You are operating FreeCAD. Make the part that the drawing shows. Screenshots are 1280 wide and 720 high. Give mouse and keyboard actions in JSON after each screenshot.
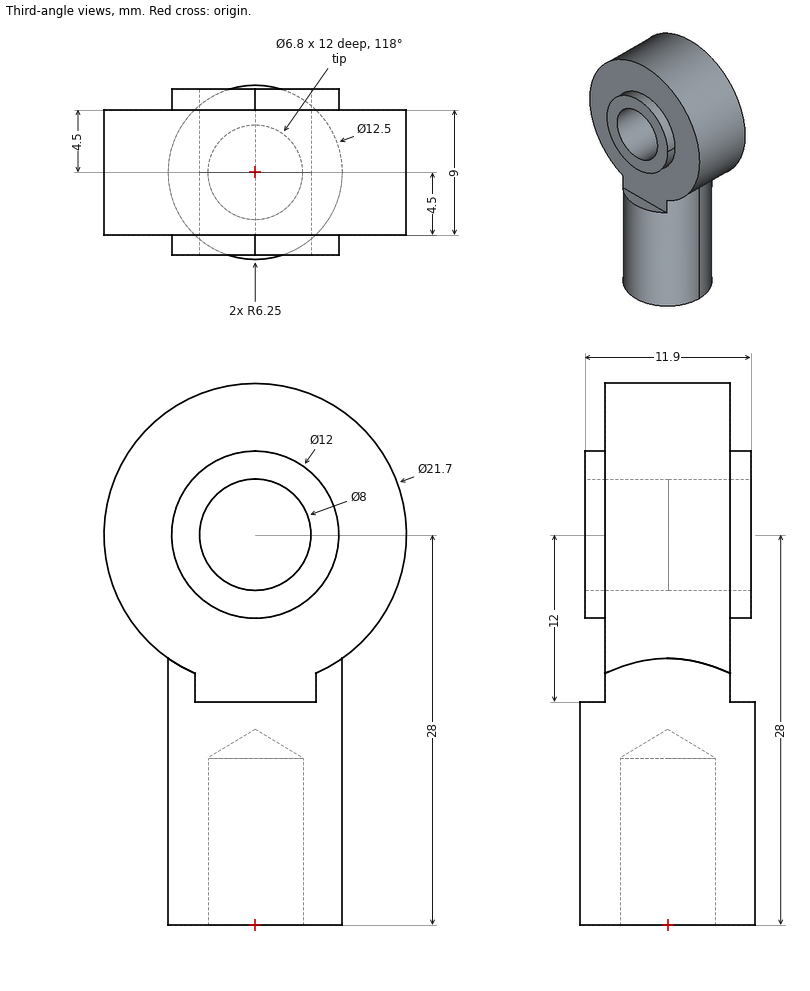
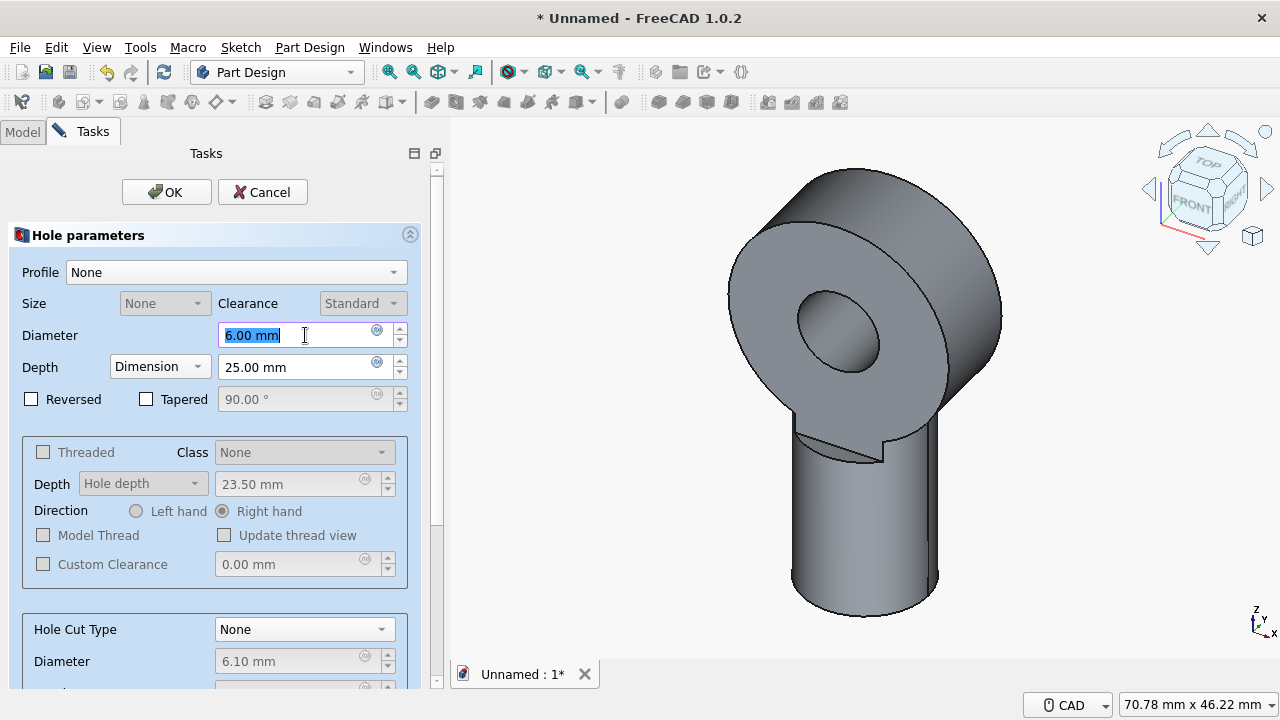
{"action": "type", "text": "6.8"}
{"action": "key", "text": "Tab"}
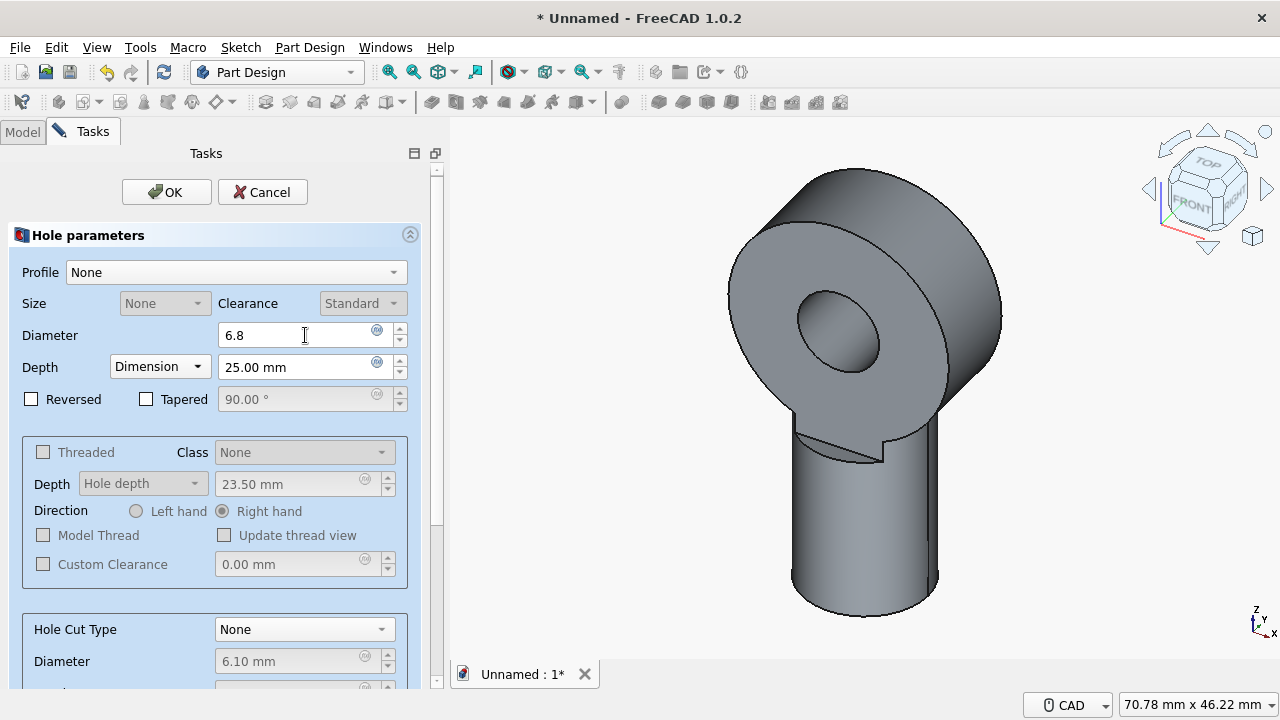
{"action": "triple_click", "coordinate": [305, 367]}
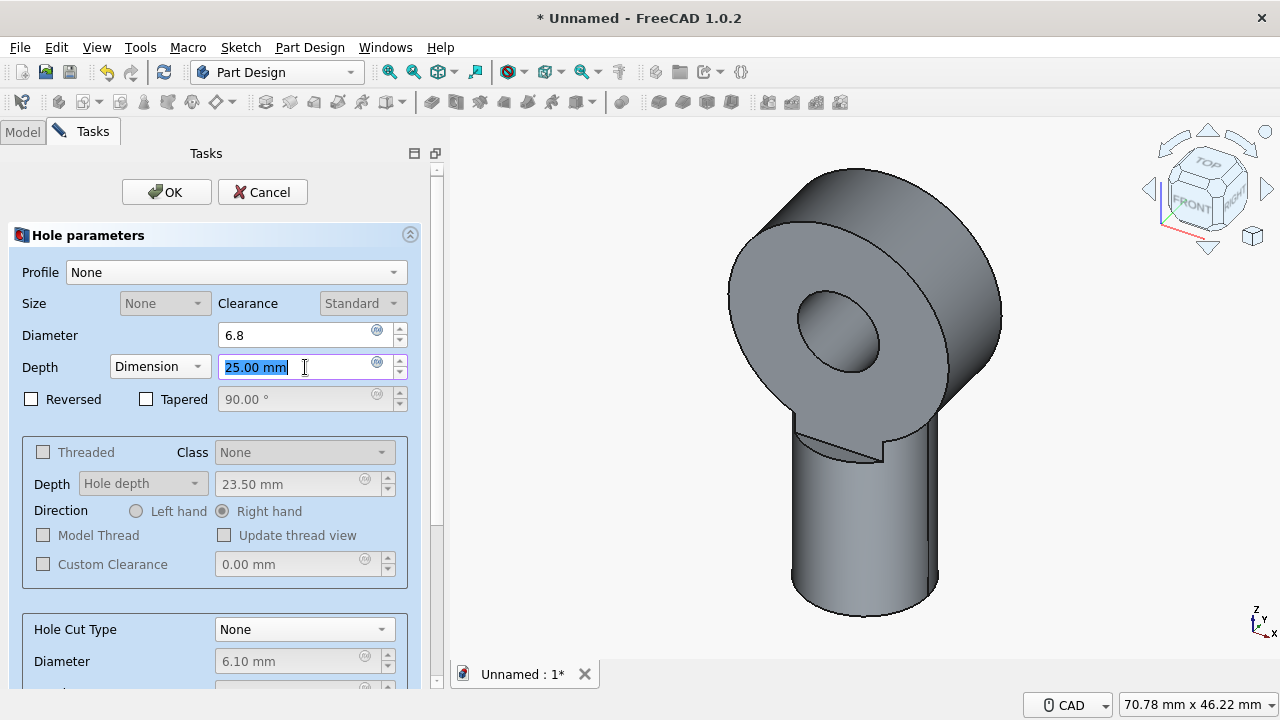
{"action": "type", "text": "12"}
{"action": "key", "text": "Tab"}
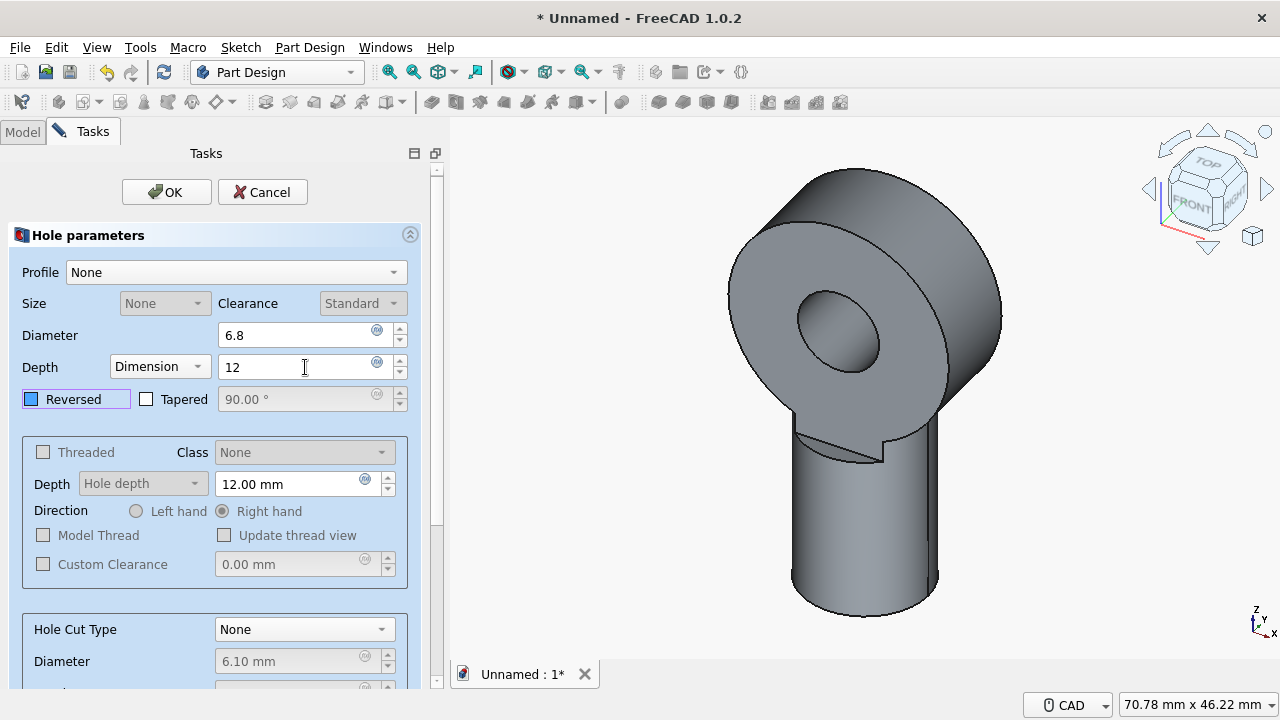
{"action": "left_click", "coordinate": [30, 399]}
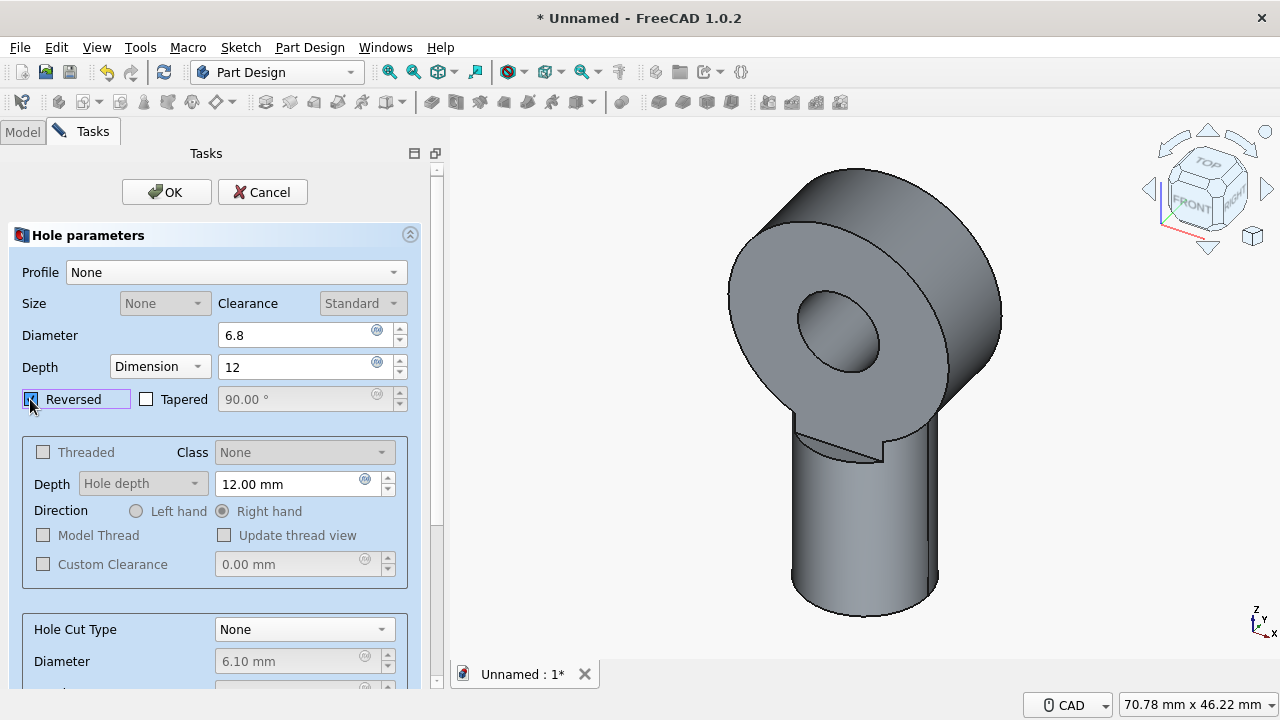
{"action": "left_click", "coordinate": [167, 192]}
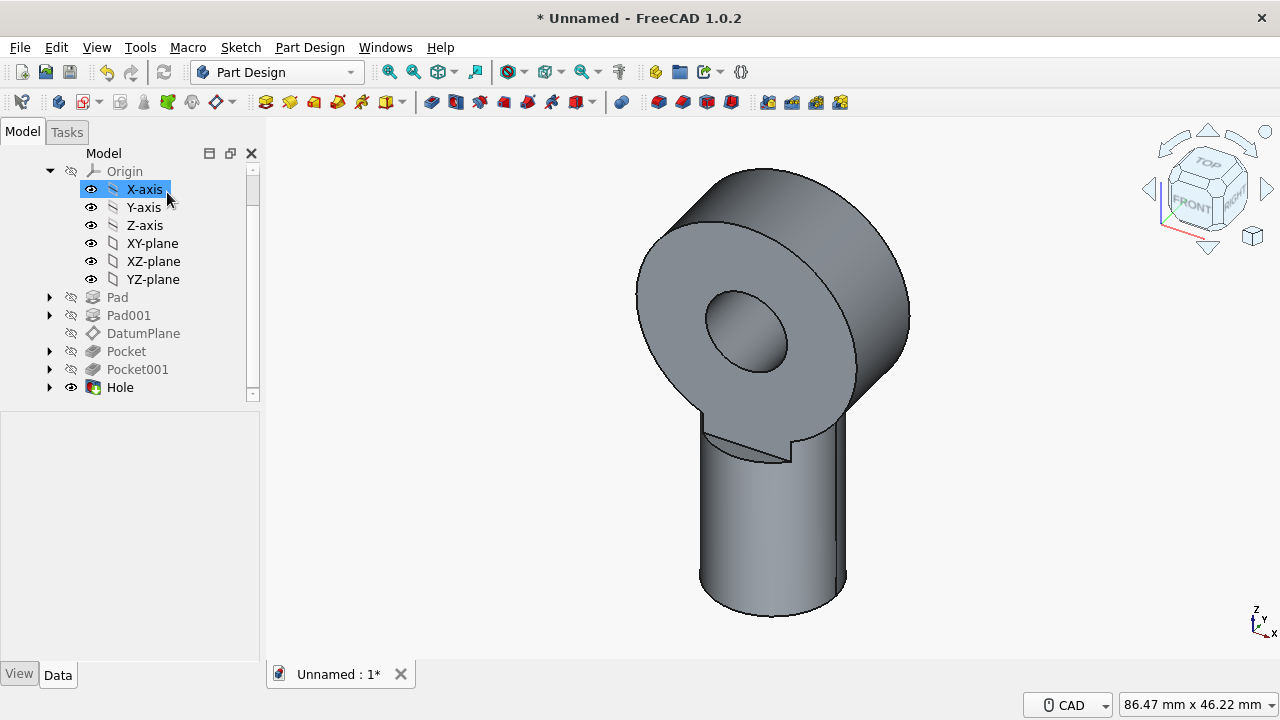
{"action": "left_click", "coordinate": [84, 102]}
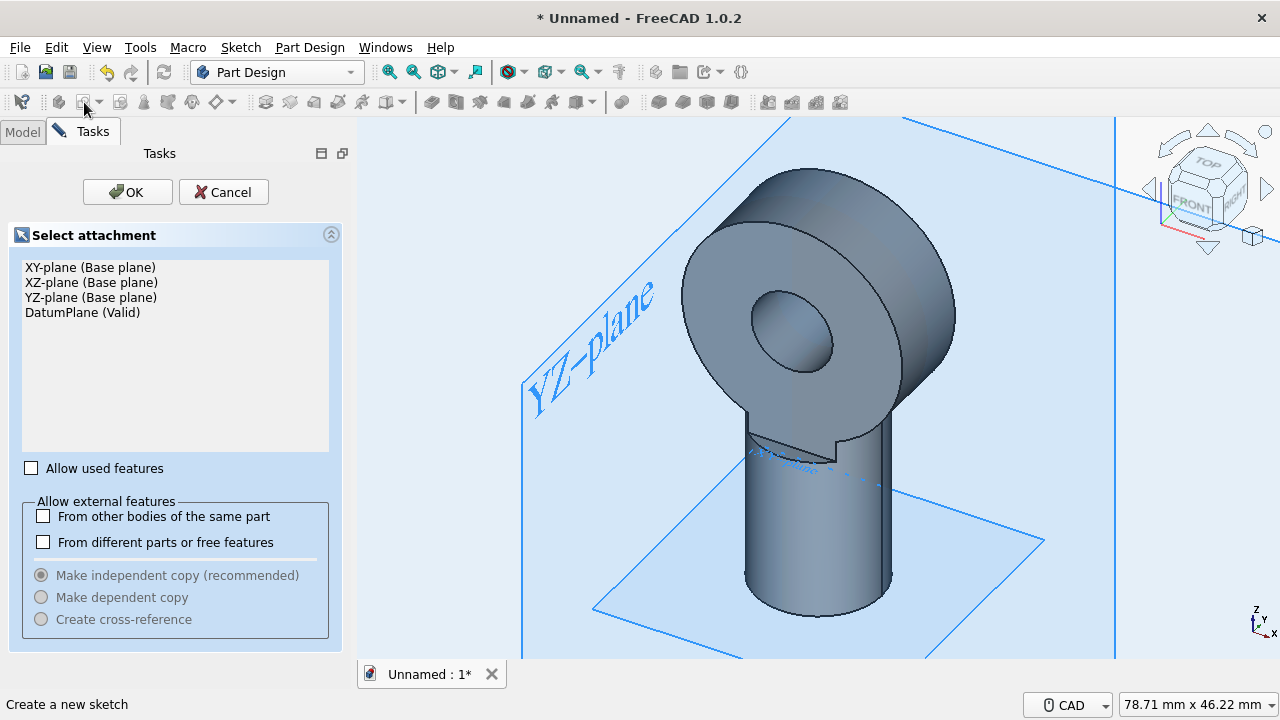
{"action": "left_click", "coordinate": [82, 282]}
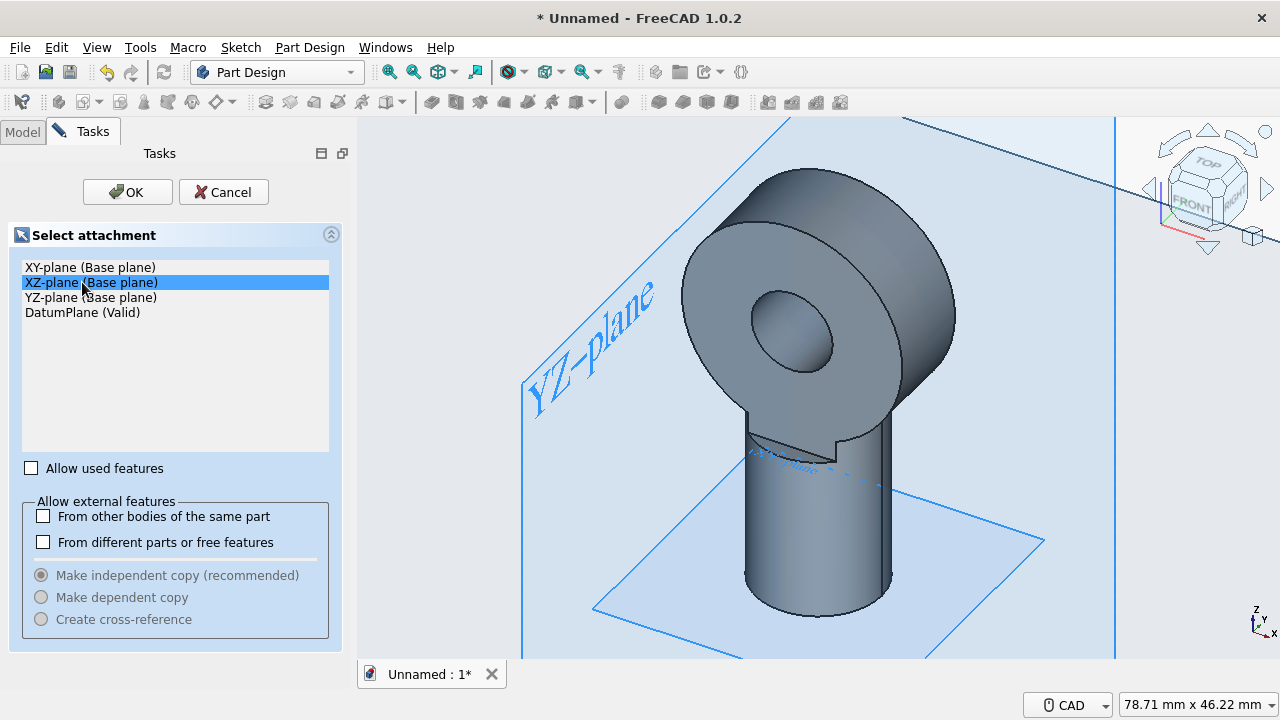
{"action": "left_click", "coordinate": [128, 192]}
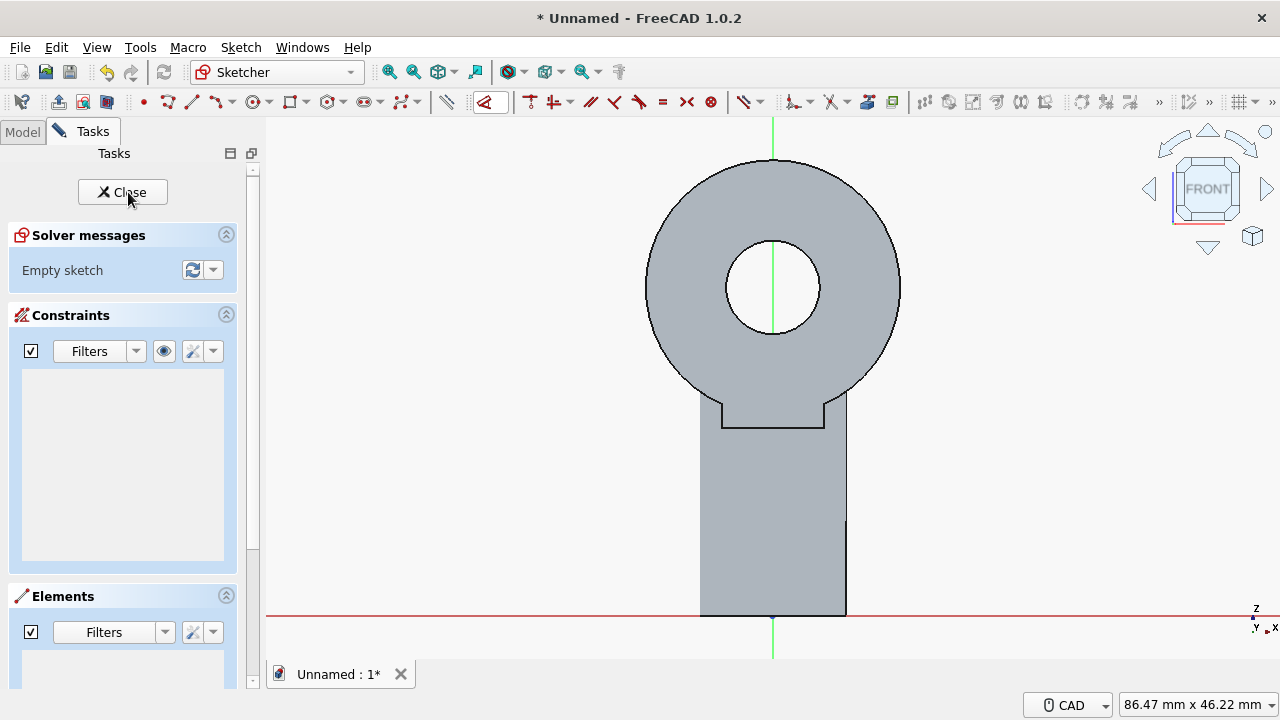
{"action": "left_click", "coordinate": [108, 102]}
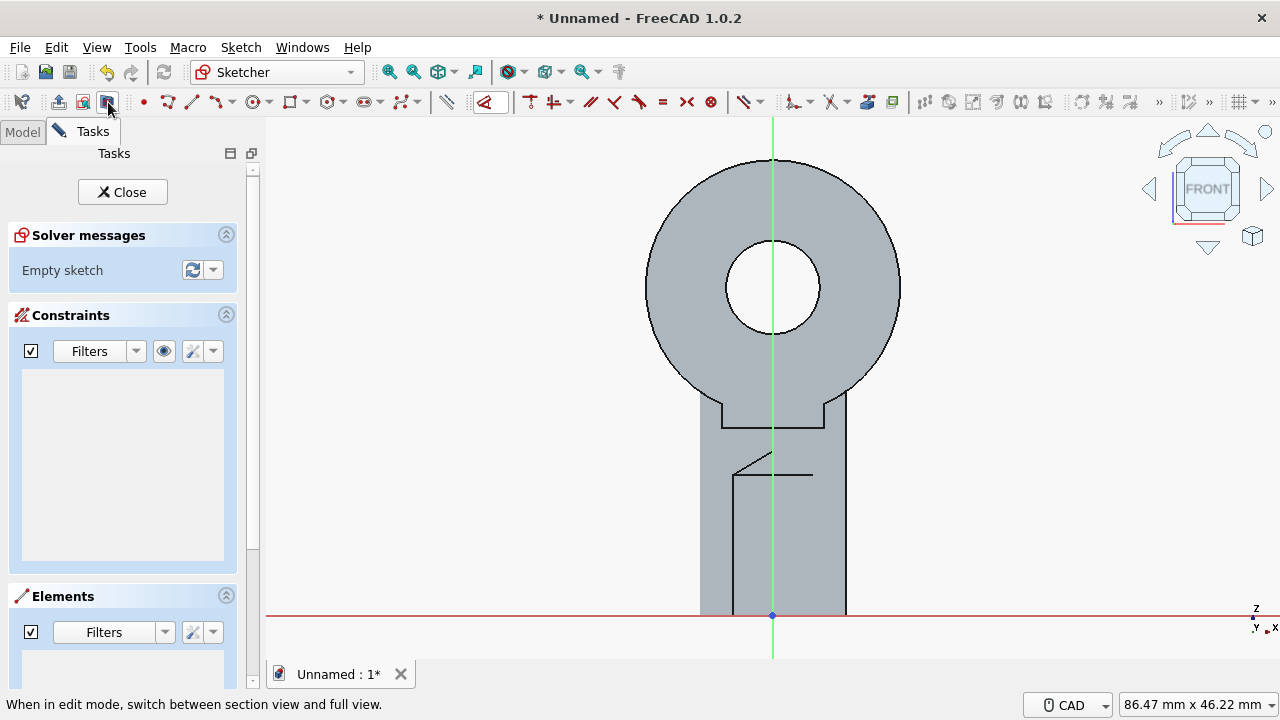
{"action": "scroll", "coordinate": [829, 205], "scroll_direction": "up", "scroll_amount": 4}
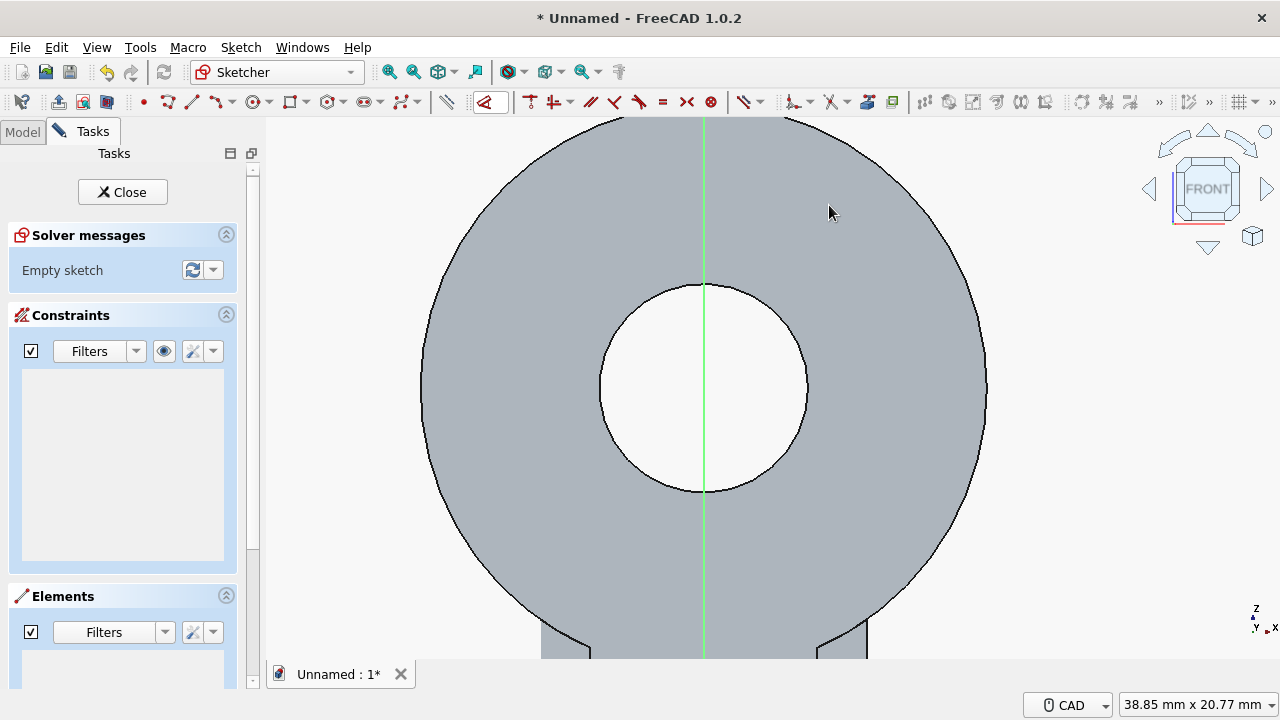
{"action": "key", "text": "g c"}